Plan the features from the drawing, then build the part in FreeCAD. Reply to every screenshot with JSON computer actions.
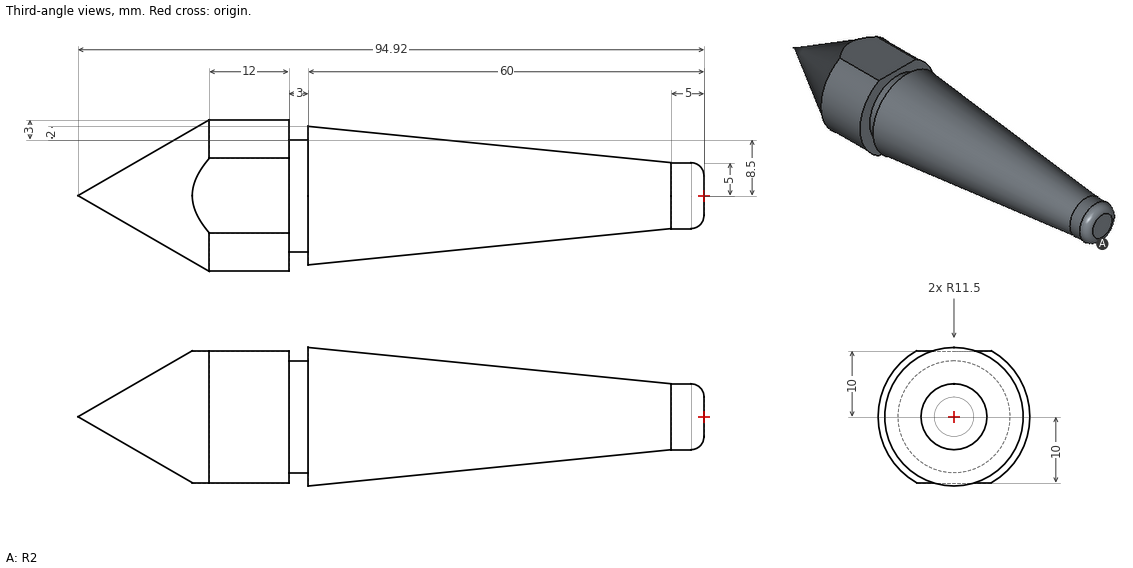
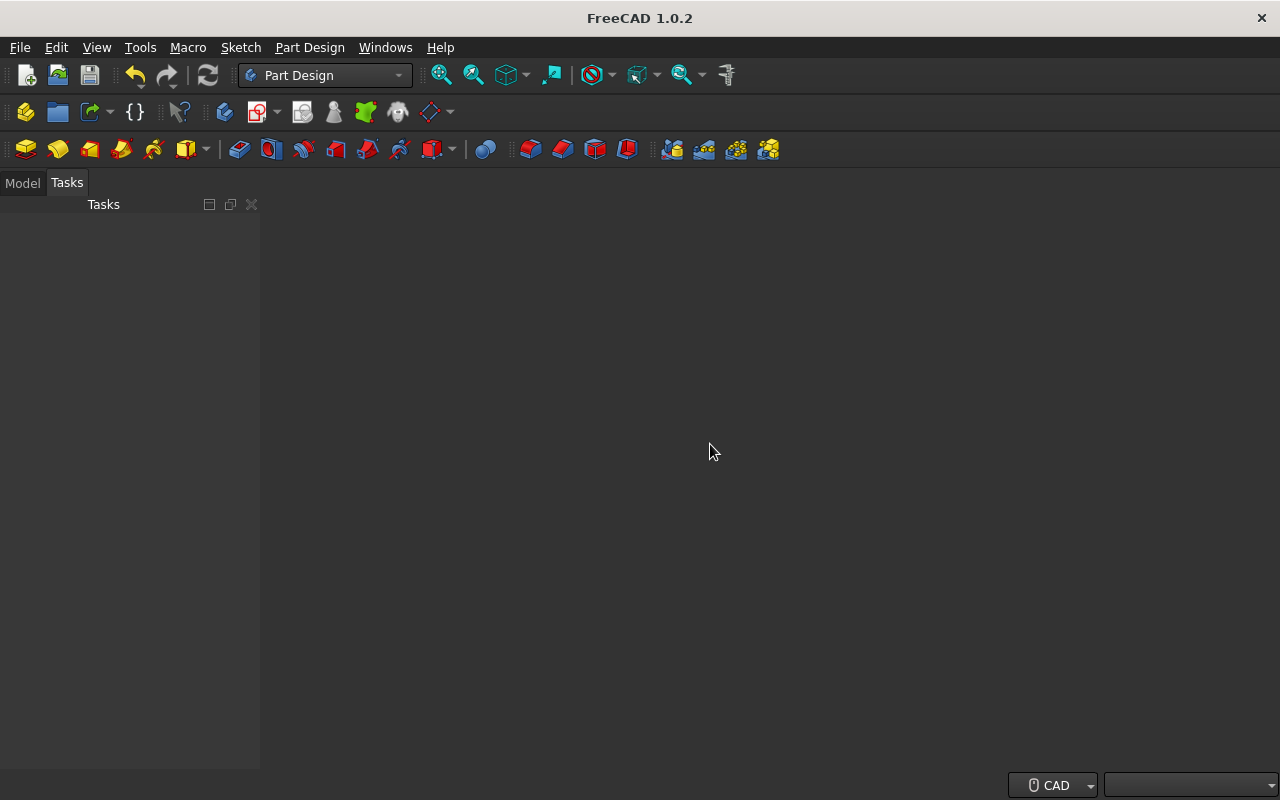
{"action": "key", "text": "ctrl+n"}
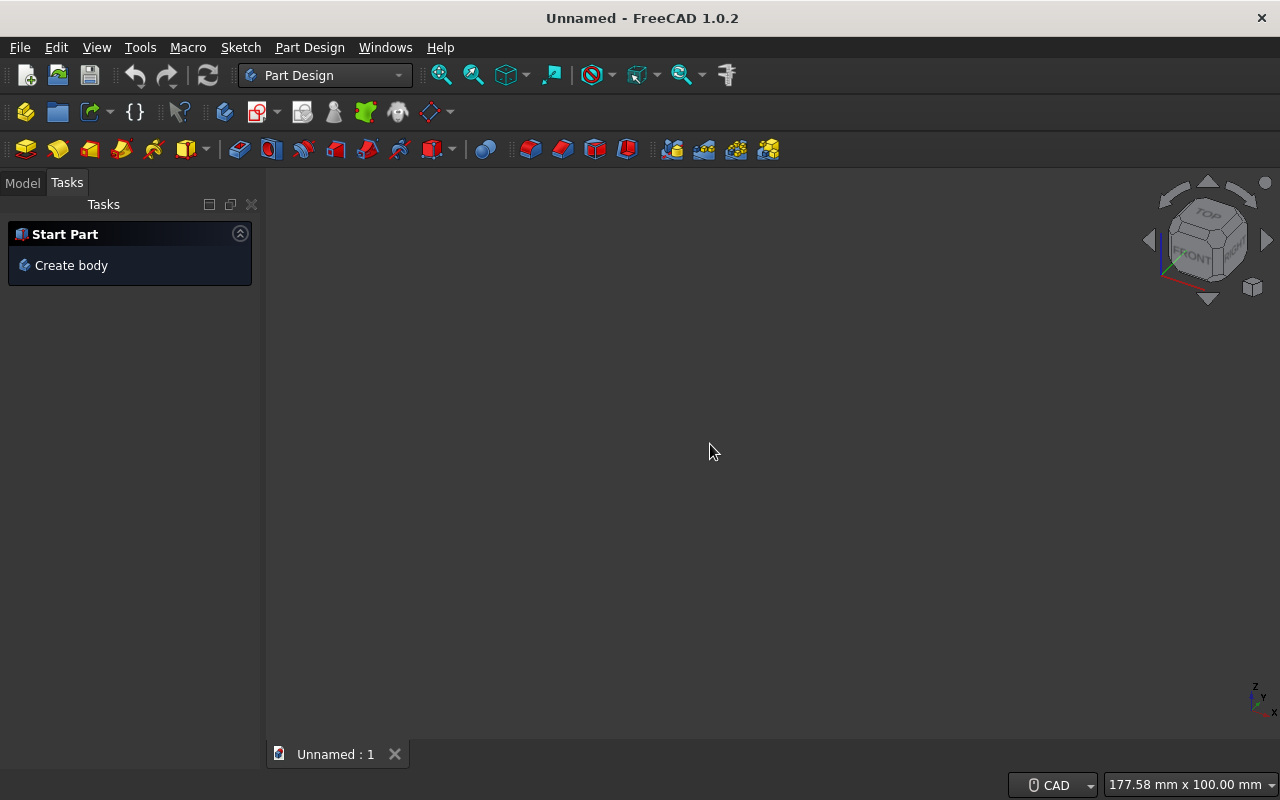
{"action": "left_click", "coordinate": [258, 112]}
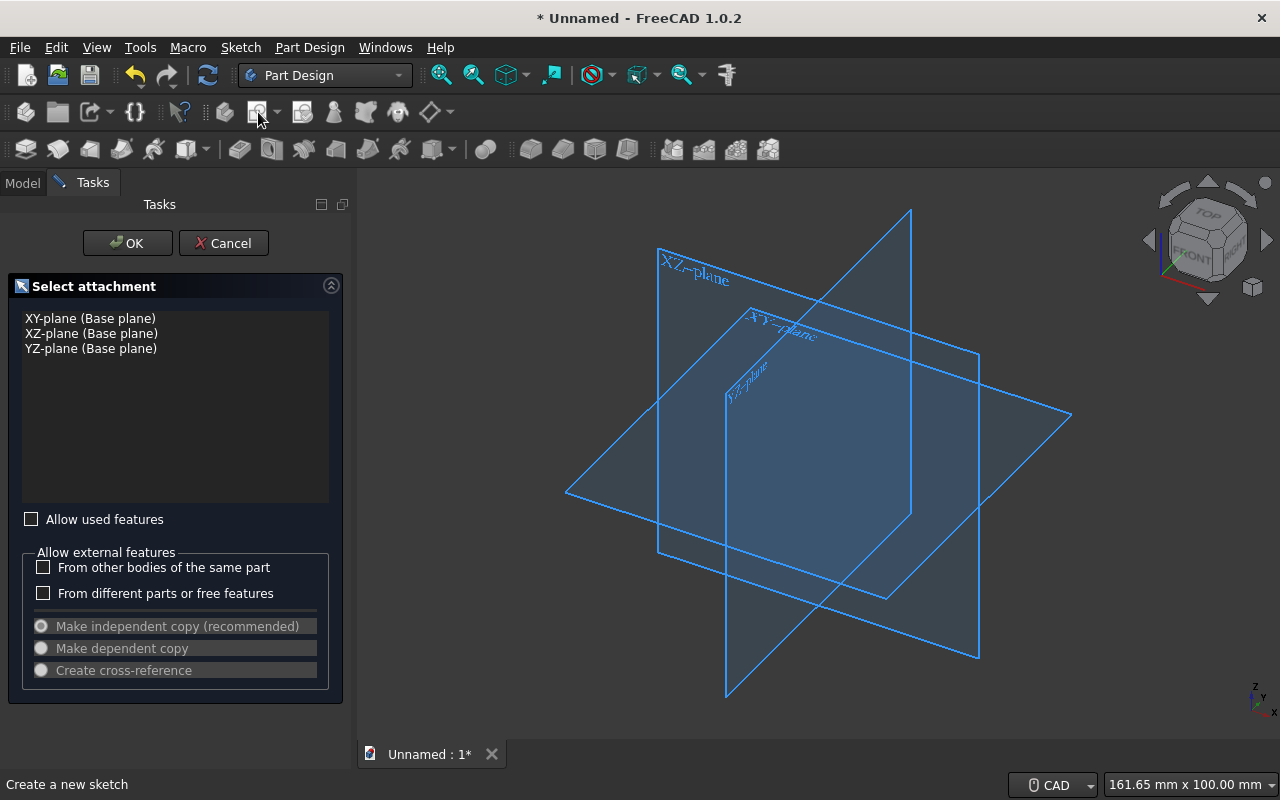
{"action": "left_click", "coordinate": [82, 318]}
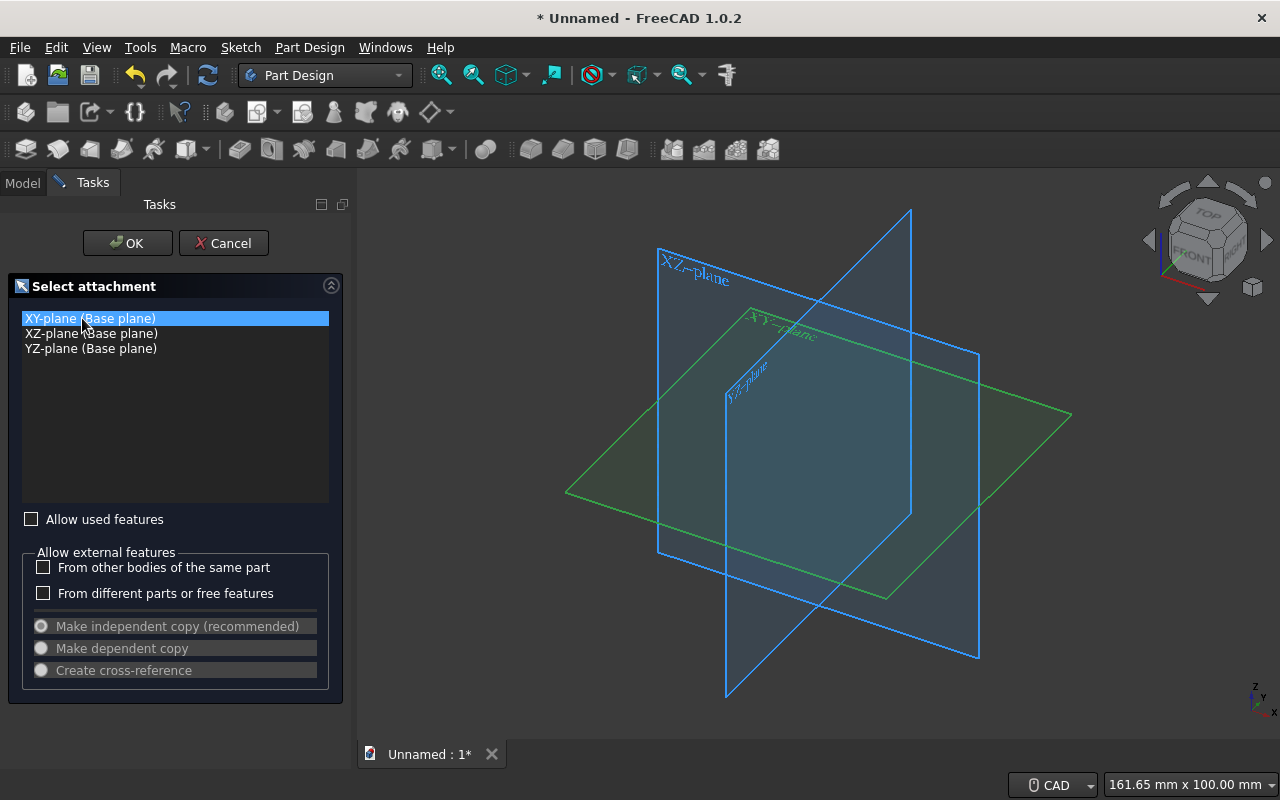
{"action": "left_click", "coordinate": [128, 243]}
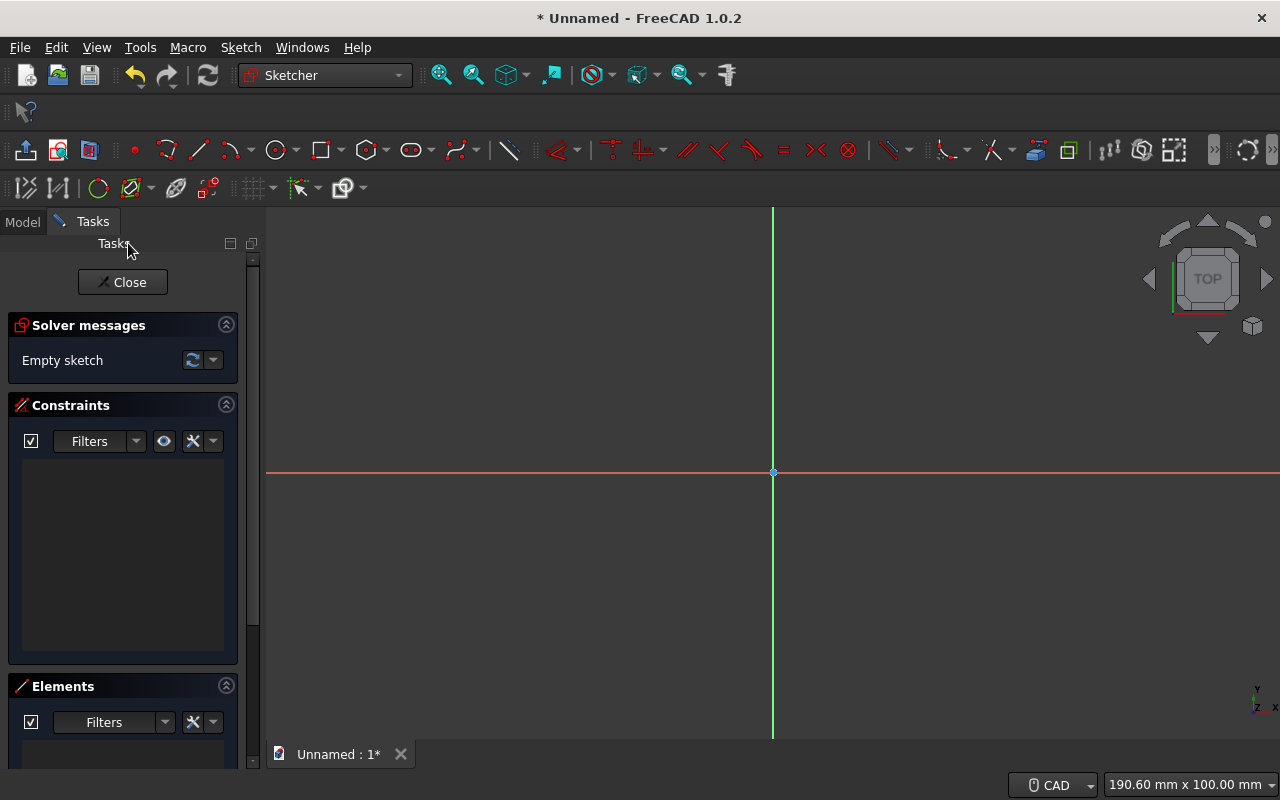
{"action": "scroll", "coordinate": [1115, 611], "scroll_direction": "down", "scroll_amount": 1}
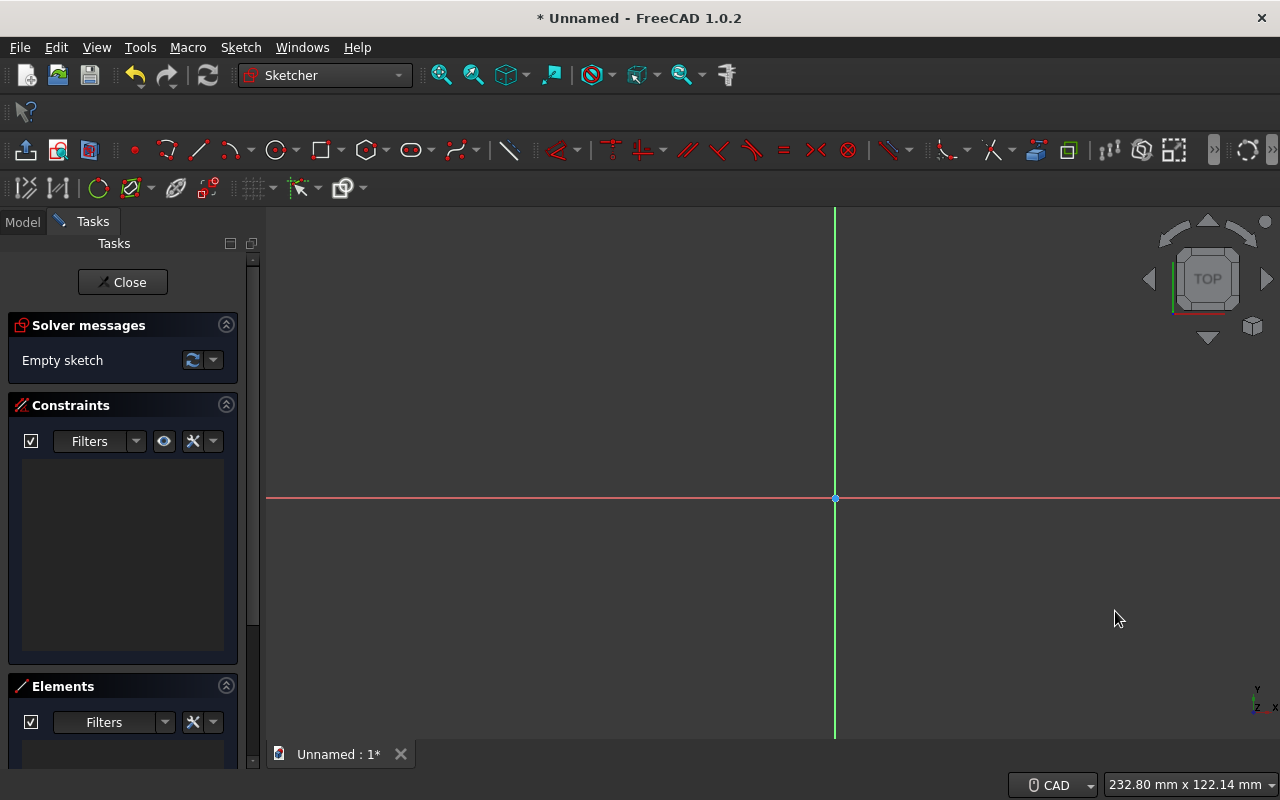
{"action": "scroll", "coordinate": [474, 473], "scroll_direction": "up", "scroll_amount": 2}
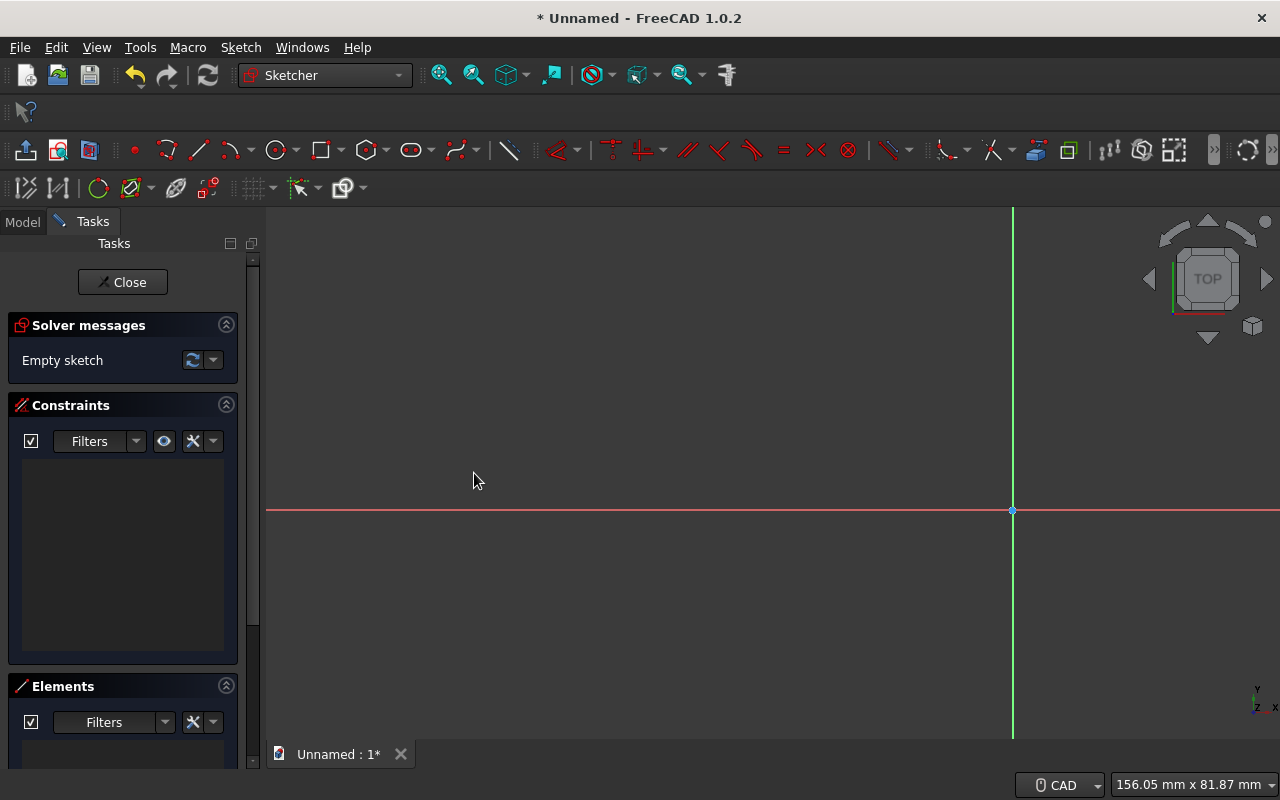
{"action": "key", "text": "g m"}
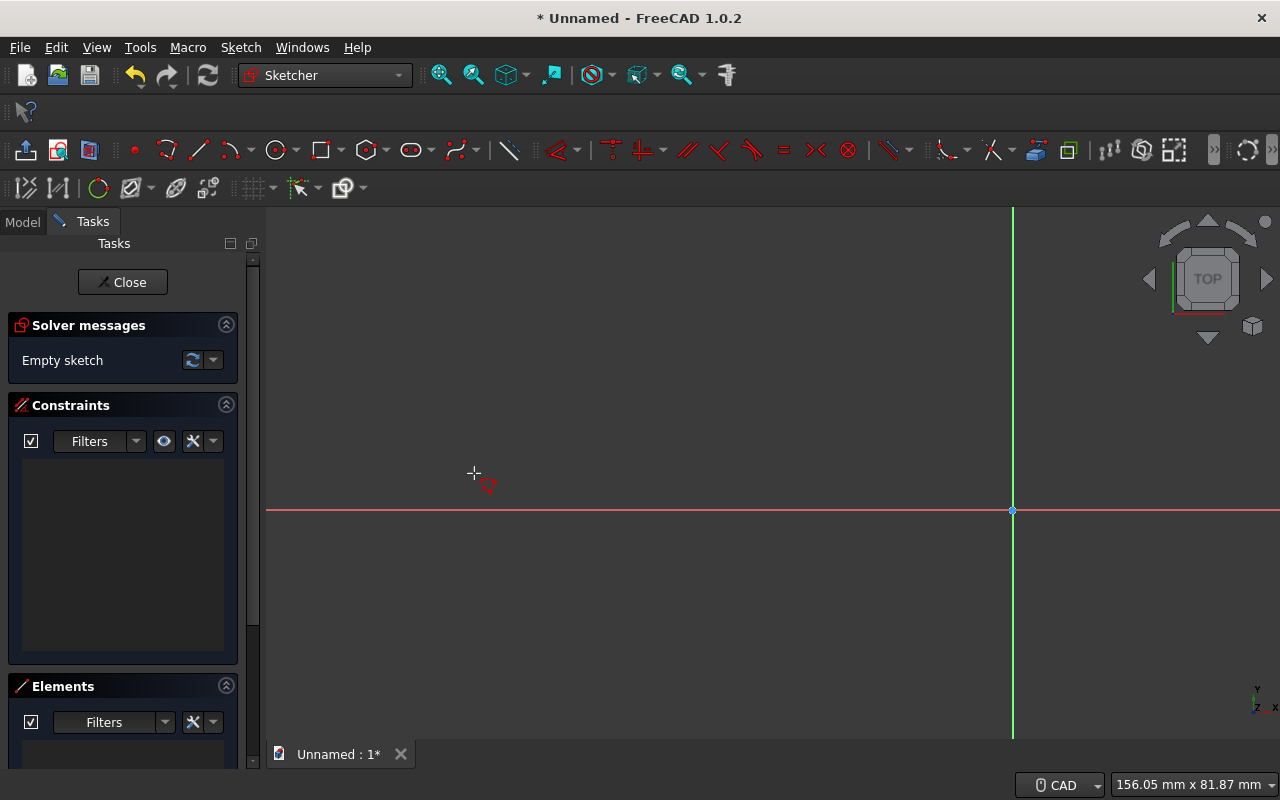
{"action": "left_click", "coordinate": [1013, 510]}
{"action": "left_click", "coordinate": [1004, 478]}
{"action": "left_click", "coordinate": [980, 478]}
{"action": "left_click", "coordinate": [623, 442]}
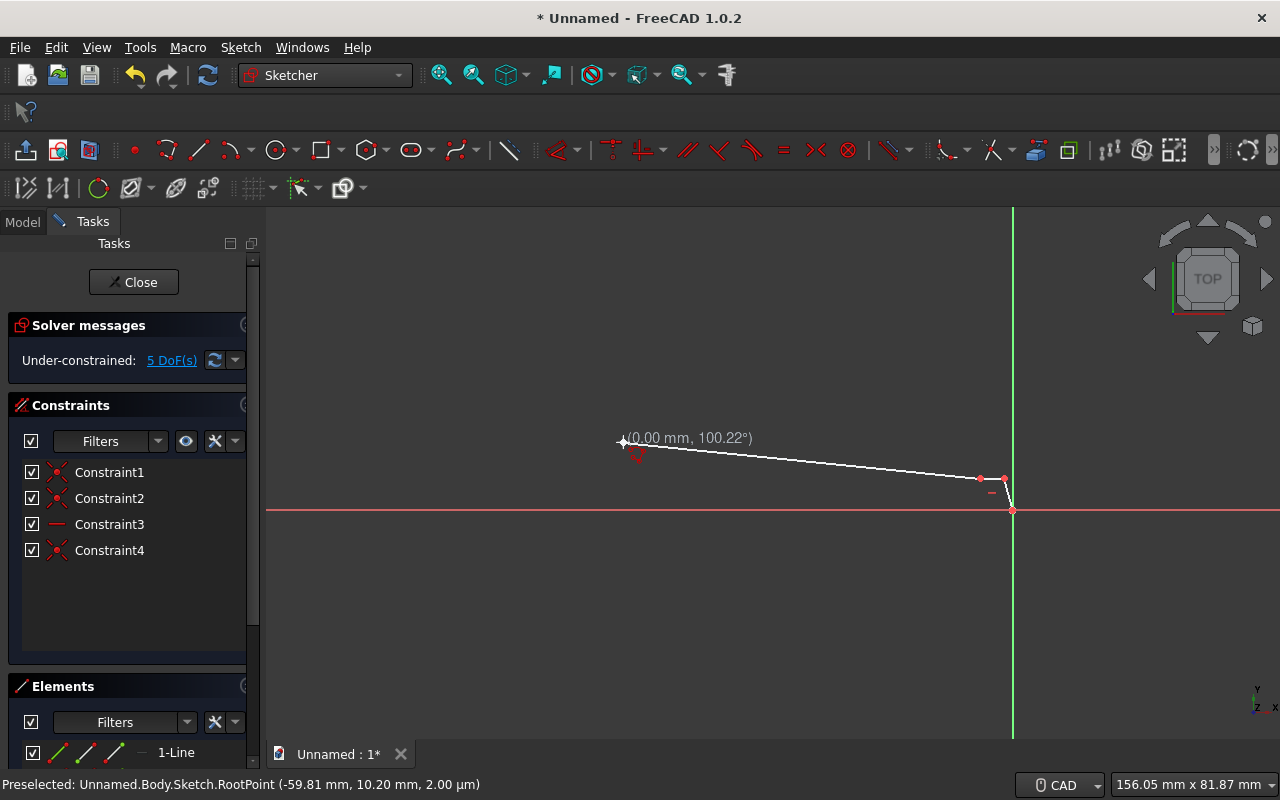
{"action": "scroll", "coordinate": [623, 455], "scroll_direction": "up", "scroll_amount": 2}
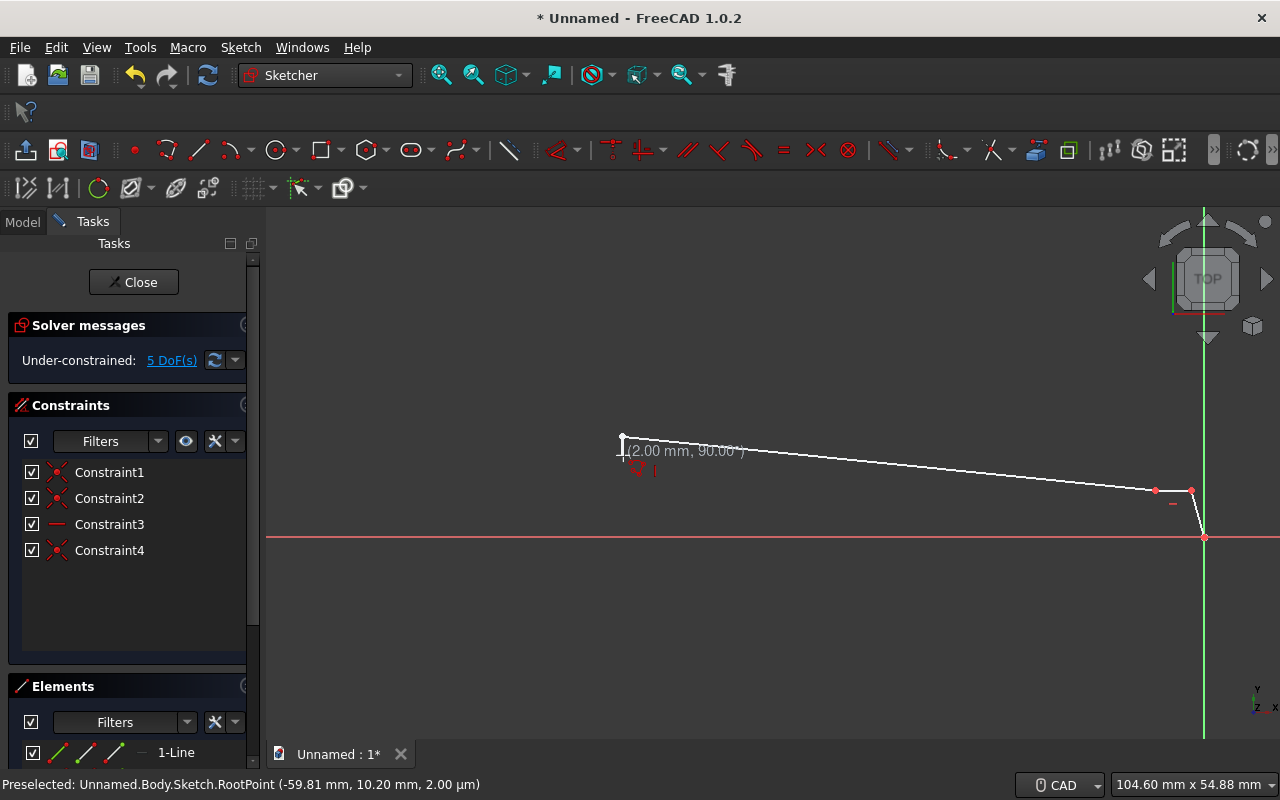
{"action": "left_click", "coordinate": [623, 455]}
{"action": "left_click", "coordinate": [593, 455]}
{"action": "left_click", "coordinate": [593, 426]}
{"action": "left_click", "coordinate": [477, 426]}